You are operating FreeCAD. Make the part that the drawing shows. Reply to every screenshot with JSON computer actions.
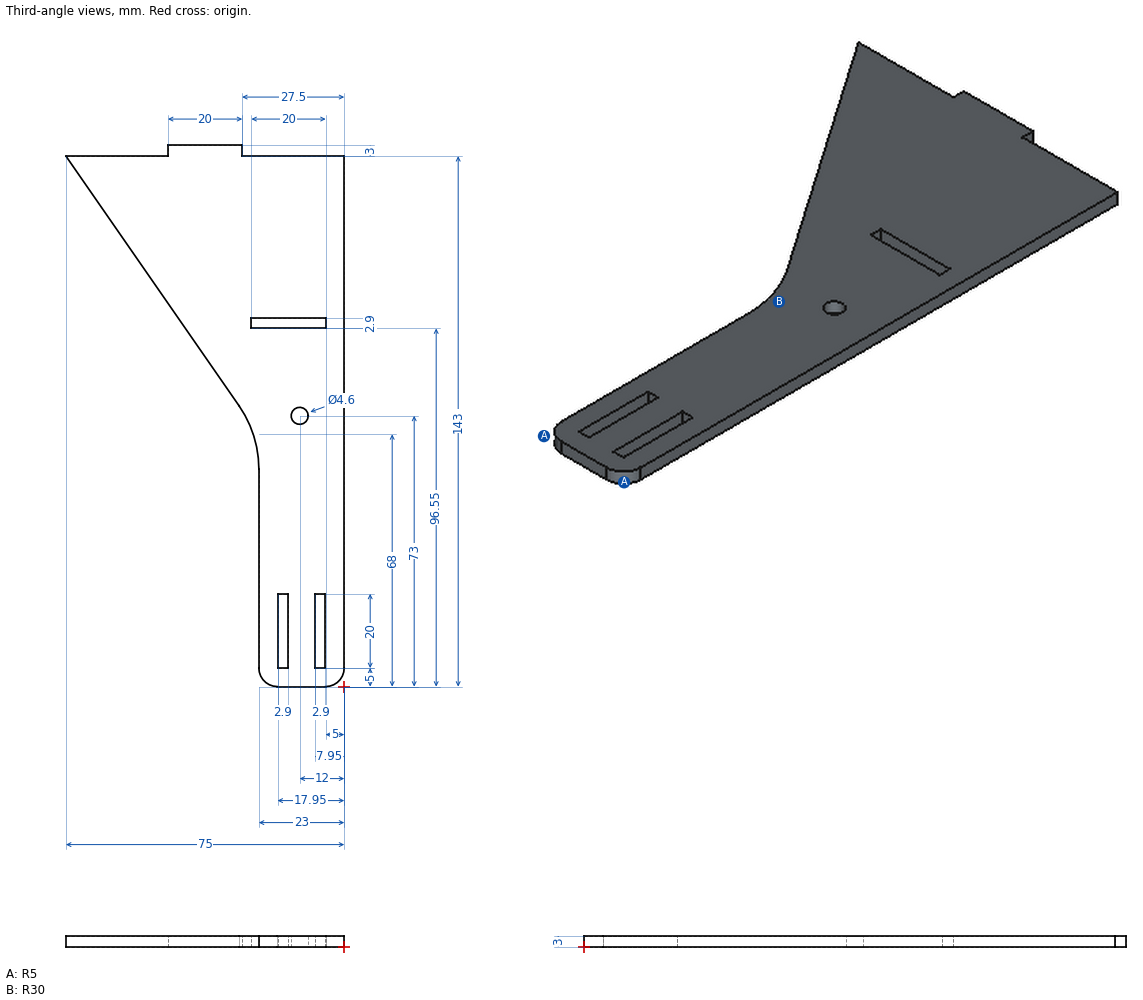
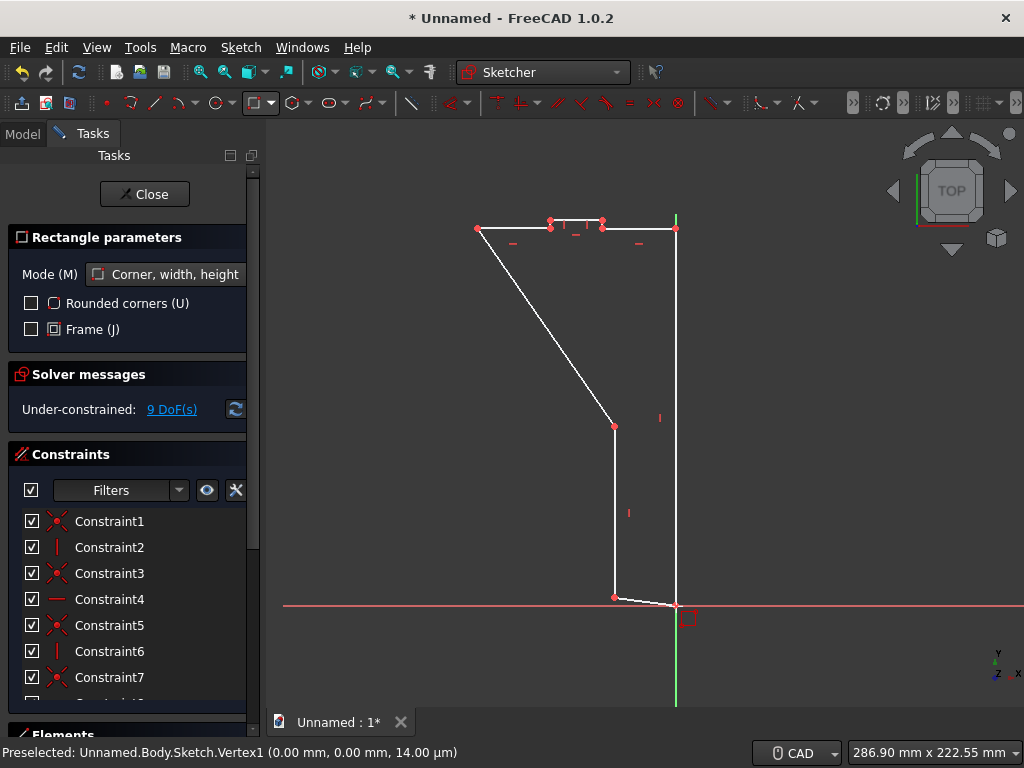
{"action": "scroll", "coordinate": [655, 540], "scroll_direction": "up", "scroll_amount": 4}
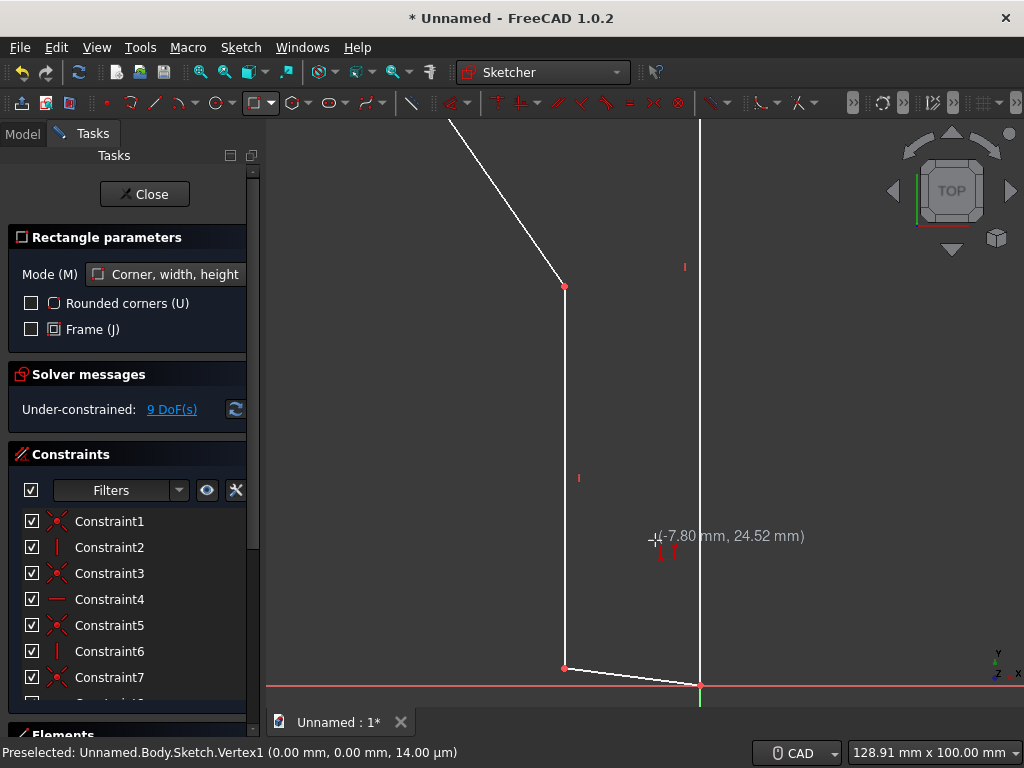
{"action": "left_click", "coordinate": [653, 539]}
{"action": "mouse_move", "coordinate": [671, 656]}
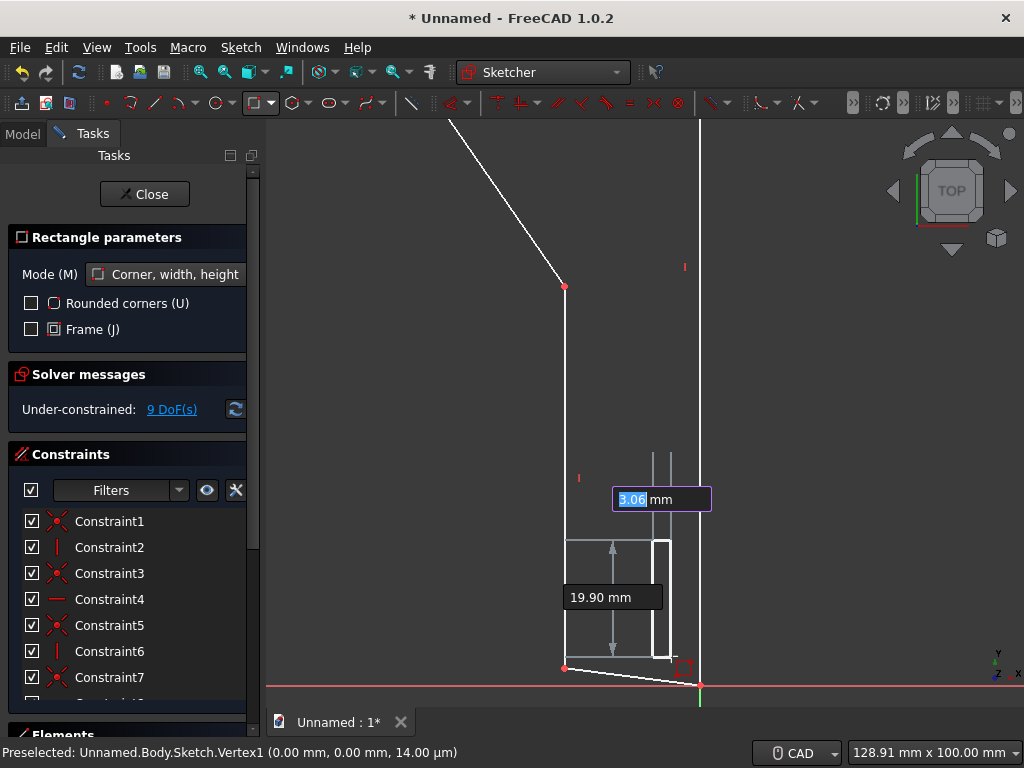
{"action": "type", "text": "2.9"}
{"action": "key", "text": "Tab"}
{"action": "type", "text": "20"}
{"action": "key", "text": "Return"}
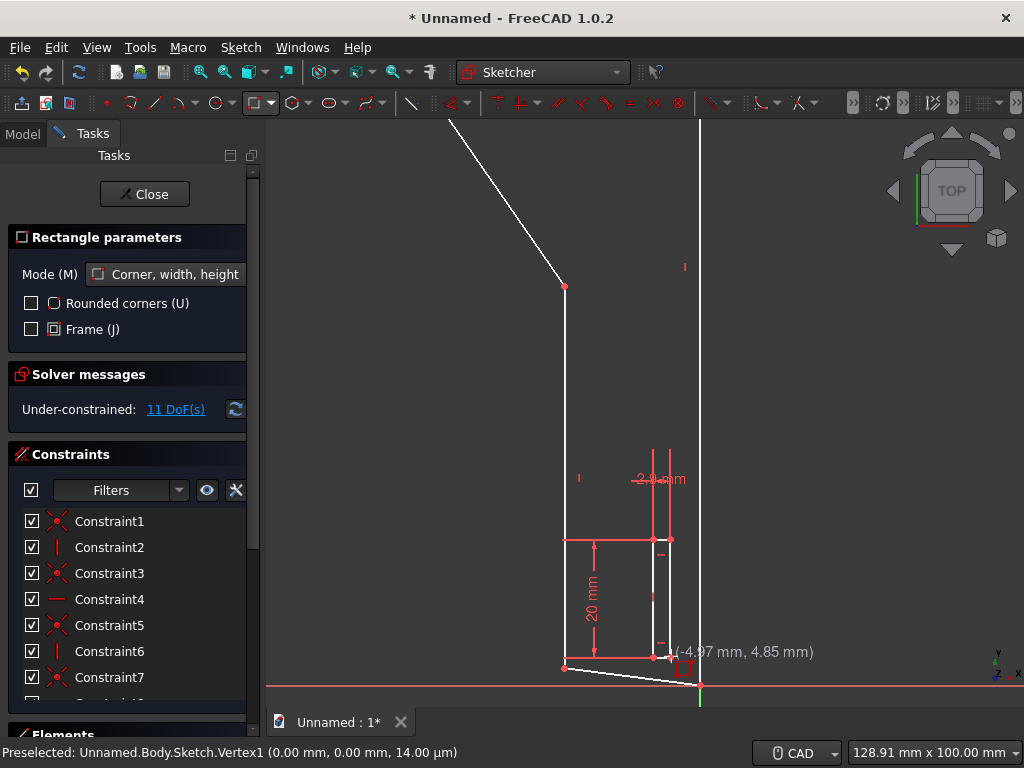
{"action": "left_click", "coordinate": [595, 539]}
{"action": "mouse_move", "coordinate": [612, 656]}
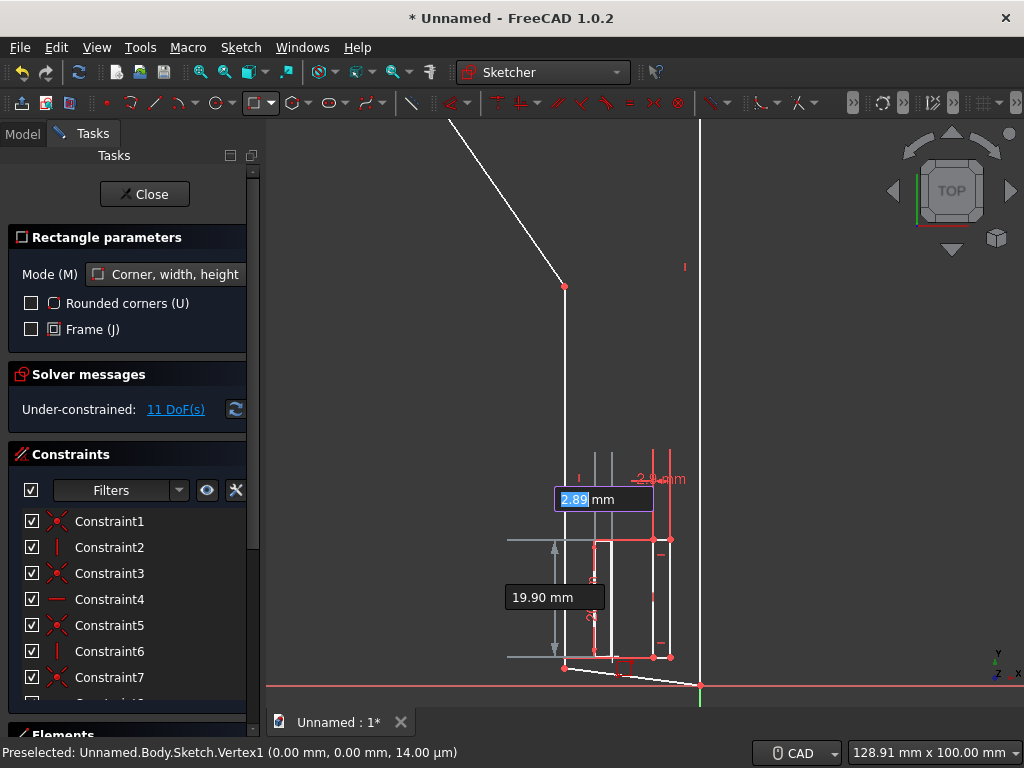
{"action": "type", "text": "2.9"}
{"action": "key", "text": "Tab"}
{"action": "type", "text": "20"}
{"action": "key", "text": "Return"}
{"action": "key", "text": "Escape"}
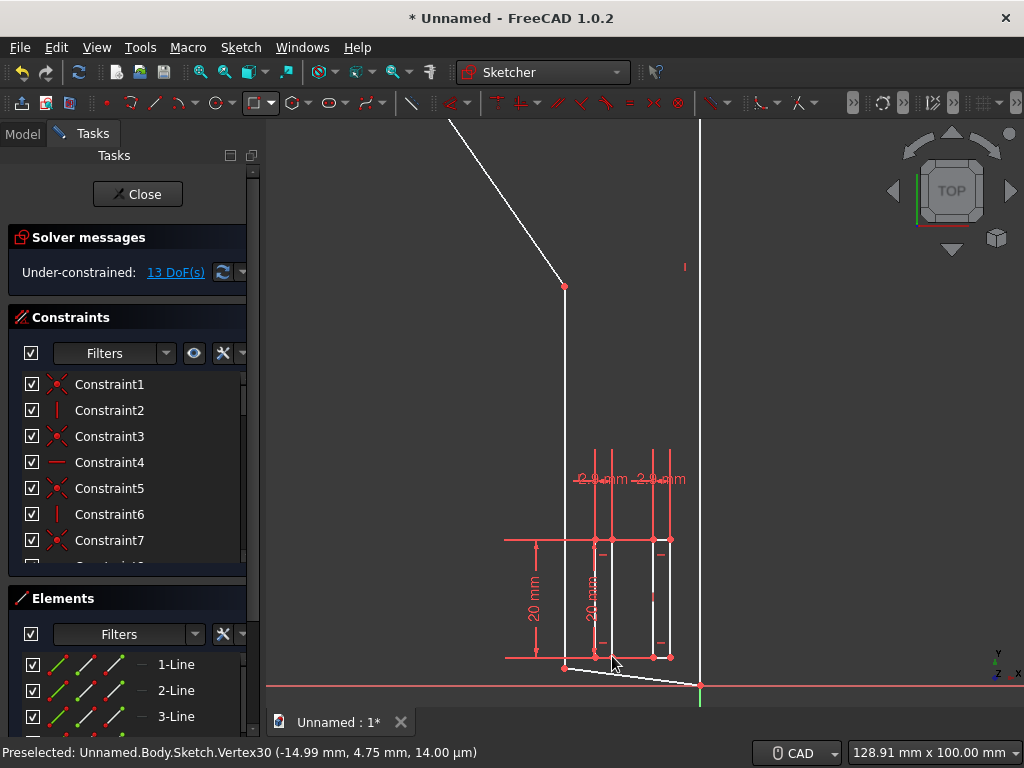
{"action": "left_click", "coordinate": [606, 673]}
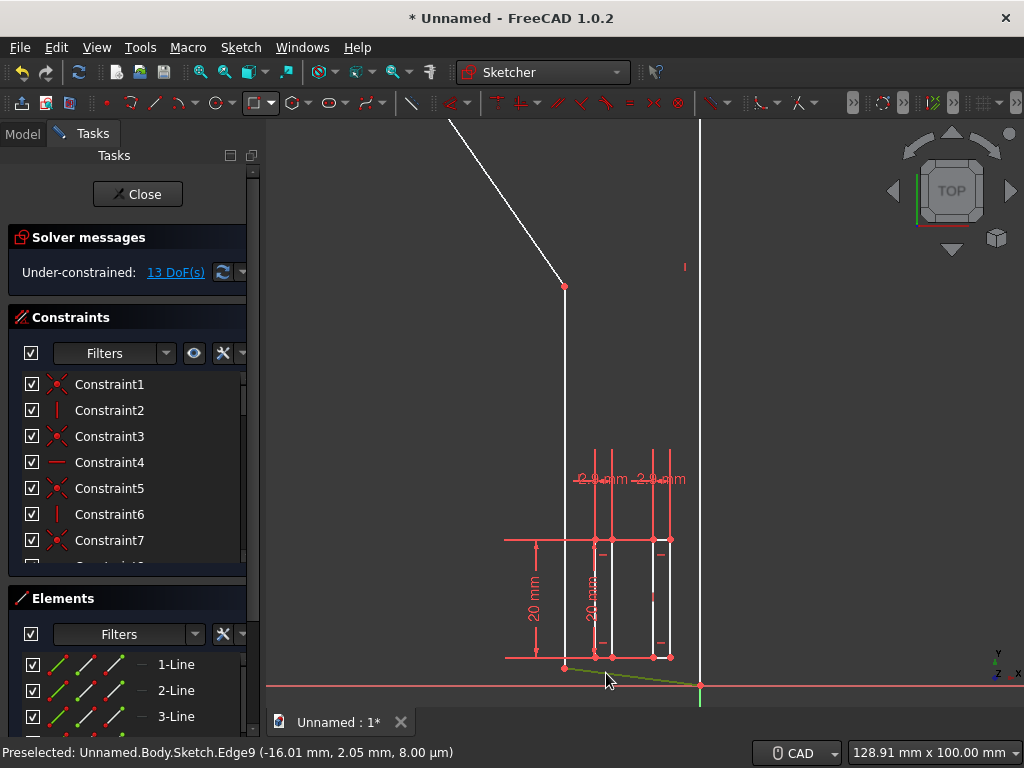
{"action": "key", "text": "h"}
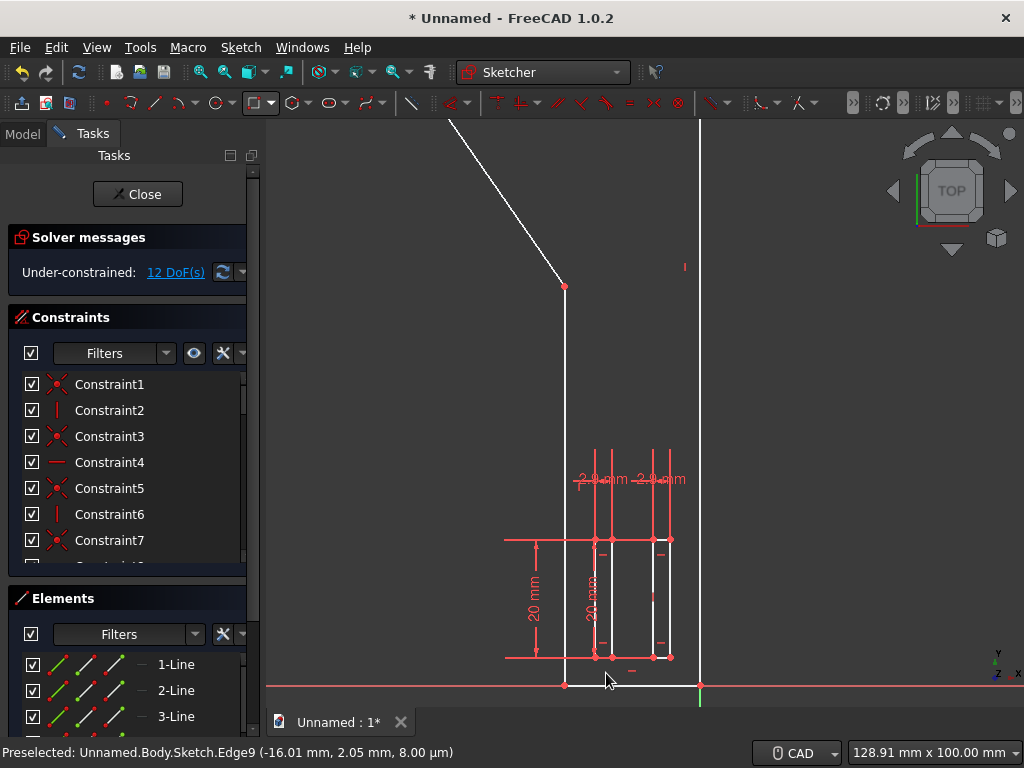
{"action": "scroll", "coordinate": [655, 541], "scroll_direction": "down", "scroll_amount": 4}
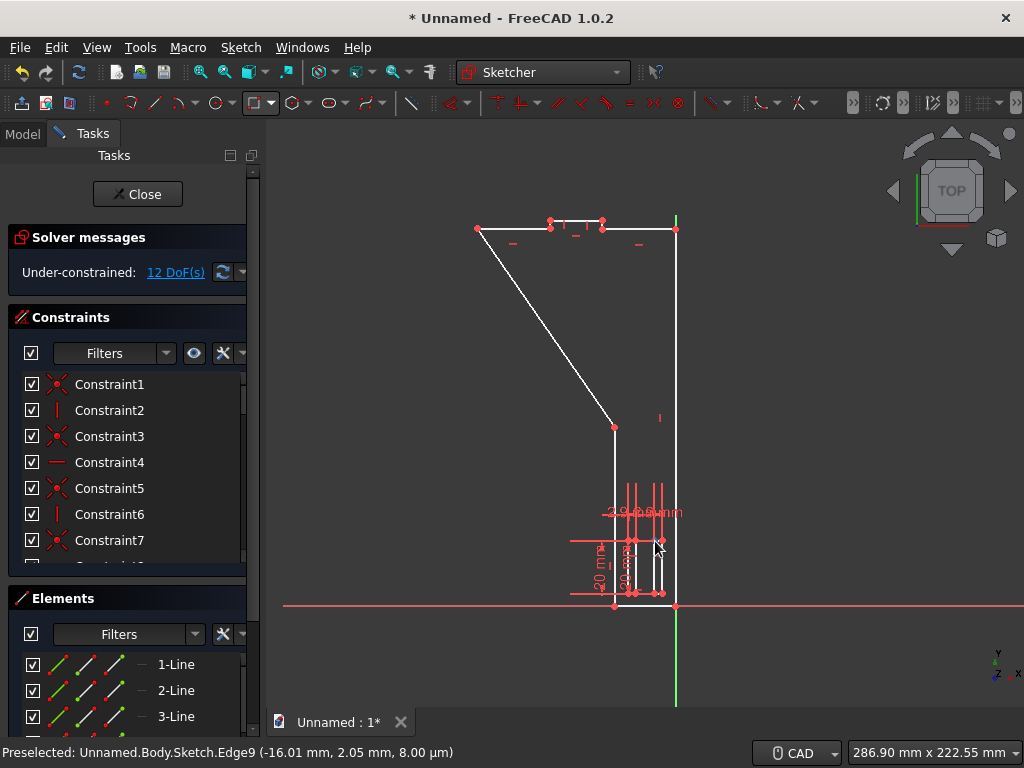
{"action": "scroll", "coordinate": [602, 225], "scroll_direction": "up", "scroll_amount": 9}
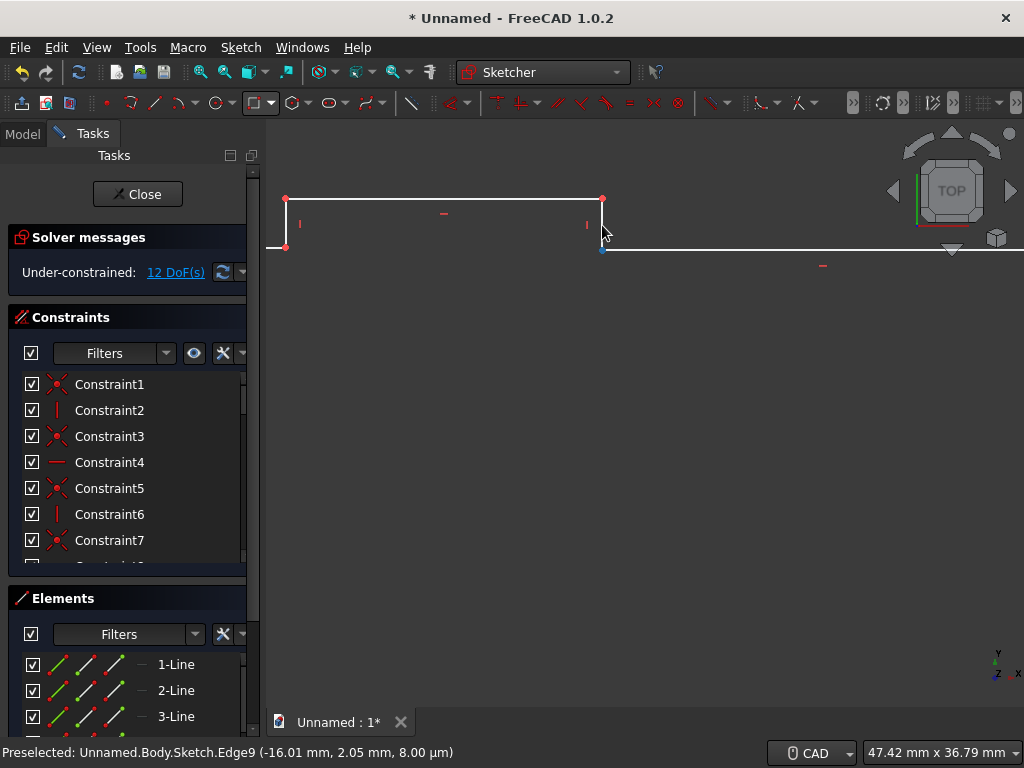
{"action": "left_click", "coordinate": [602, 225]}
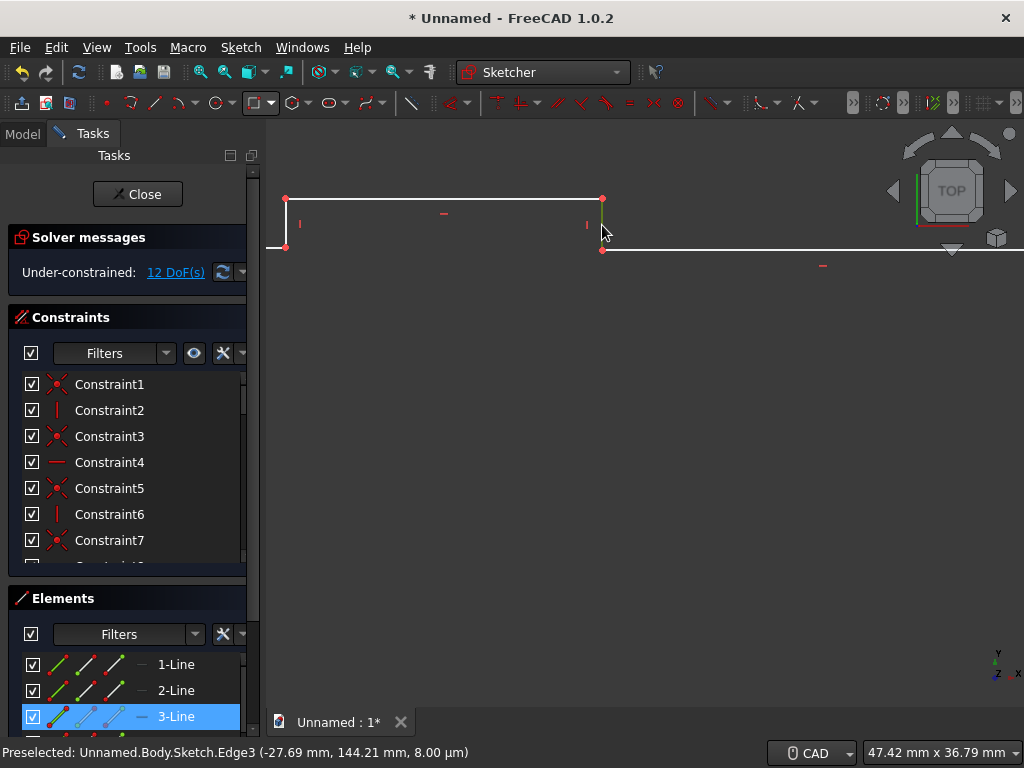
{"action": "left_click", "coordinate": [470, 104]}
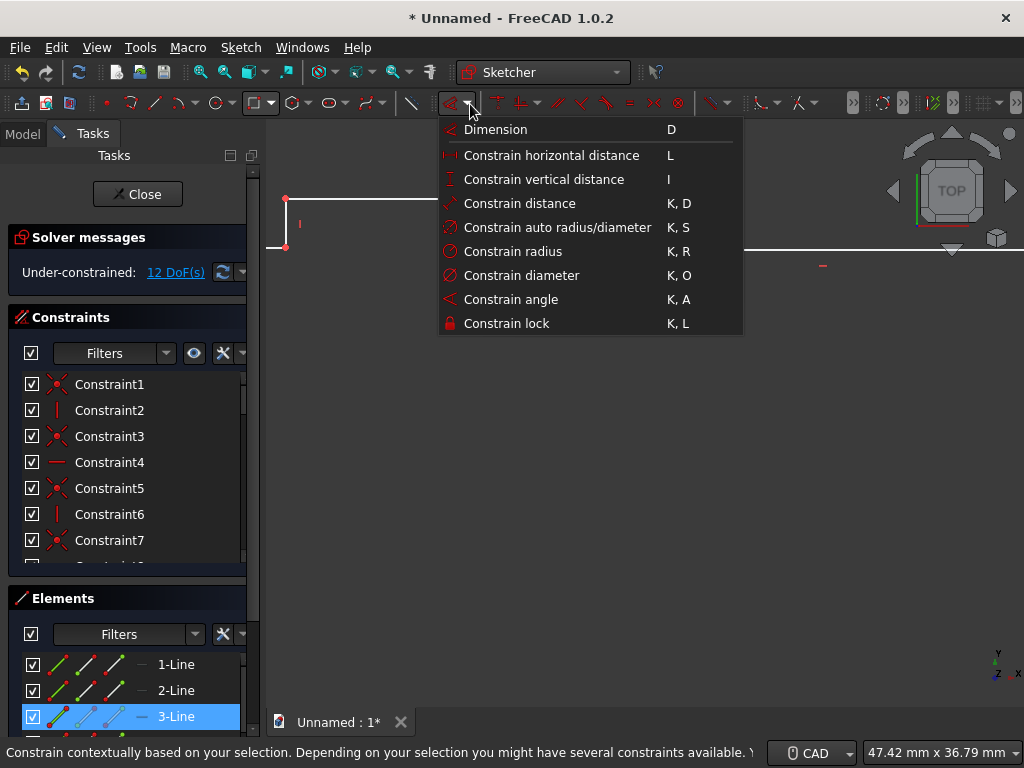
{"action": "left_click", "coordinate": [591, 179]}